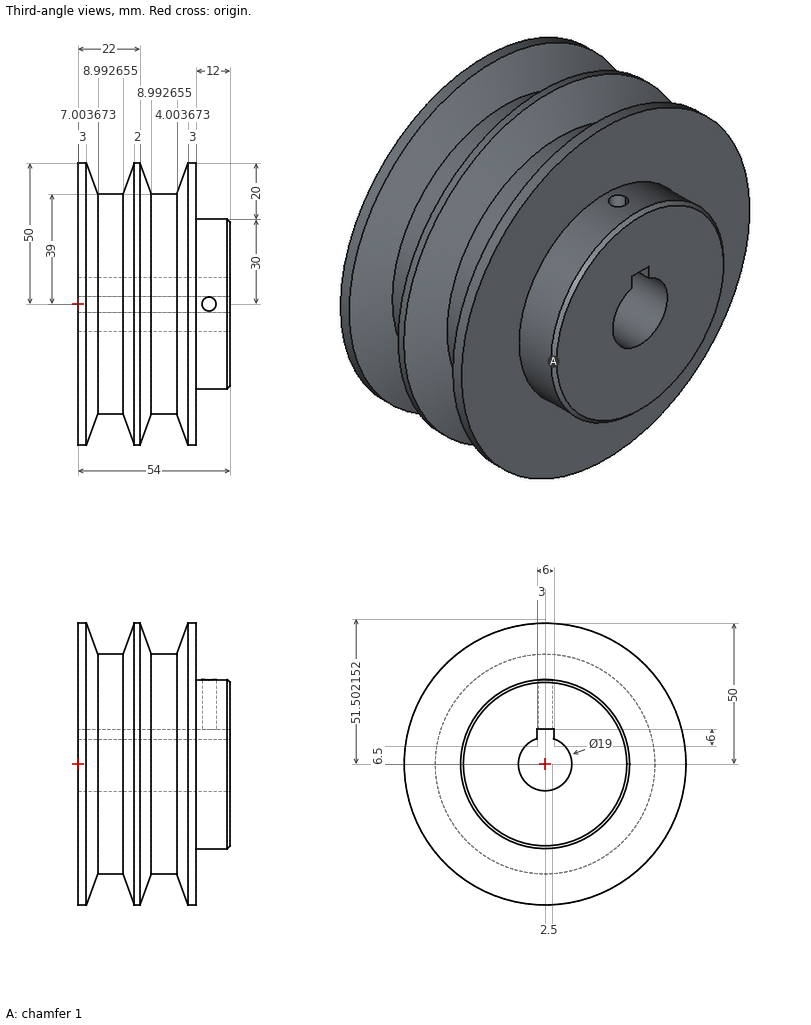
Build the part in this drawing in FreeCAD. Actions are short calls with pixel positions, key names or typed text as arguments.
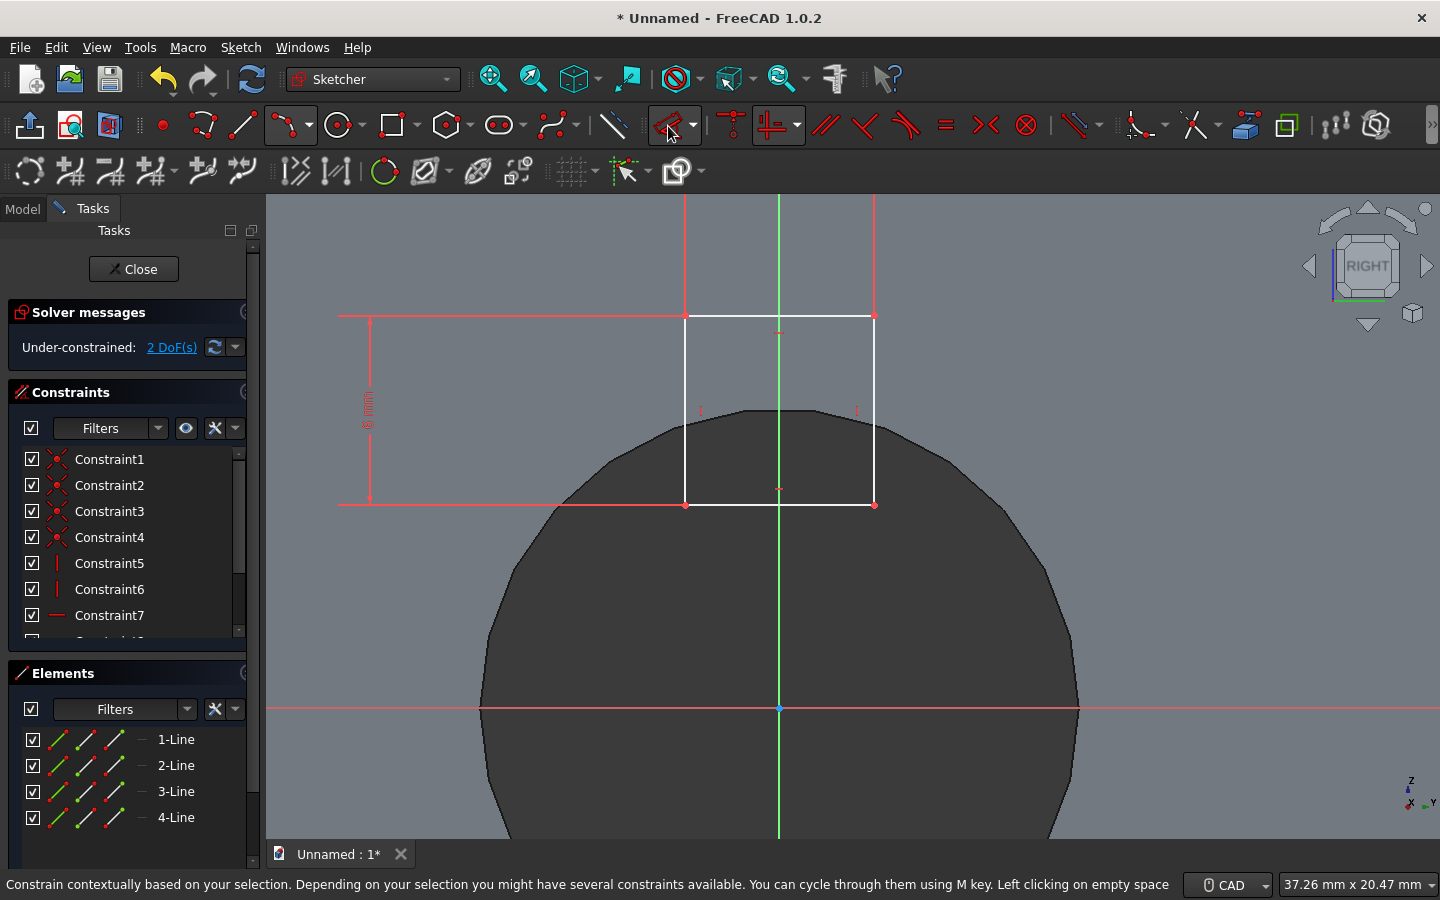
click(685, 316)
click(732, 742)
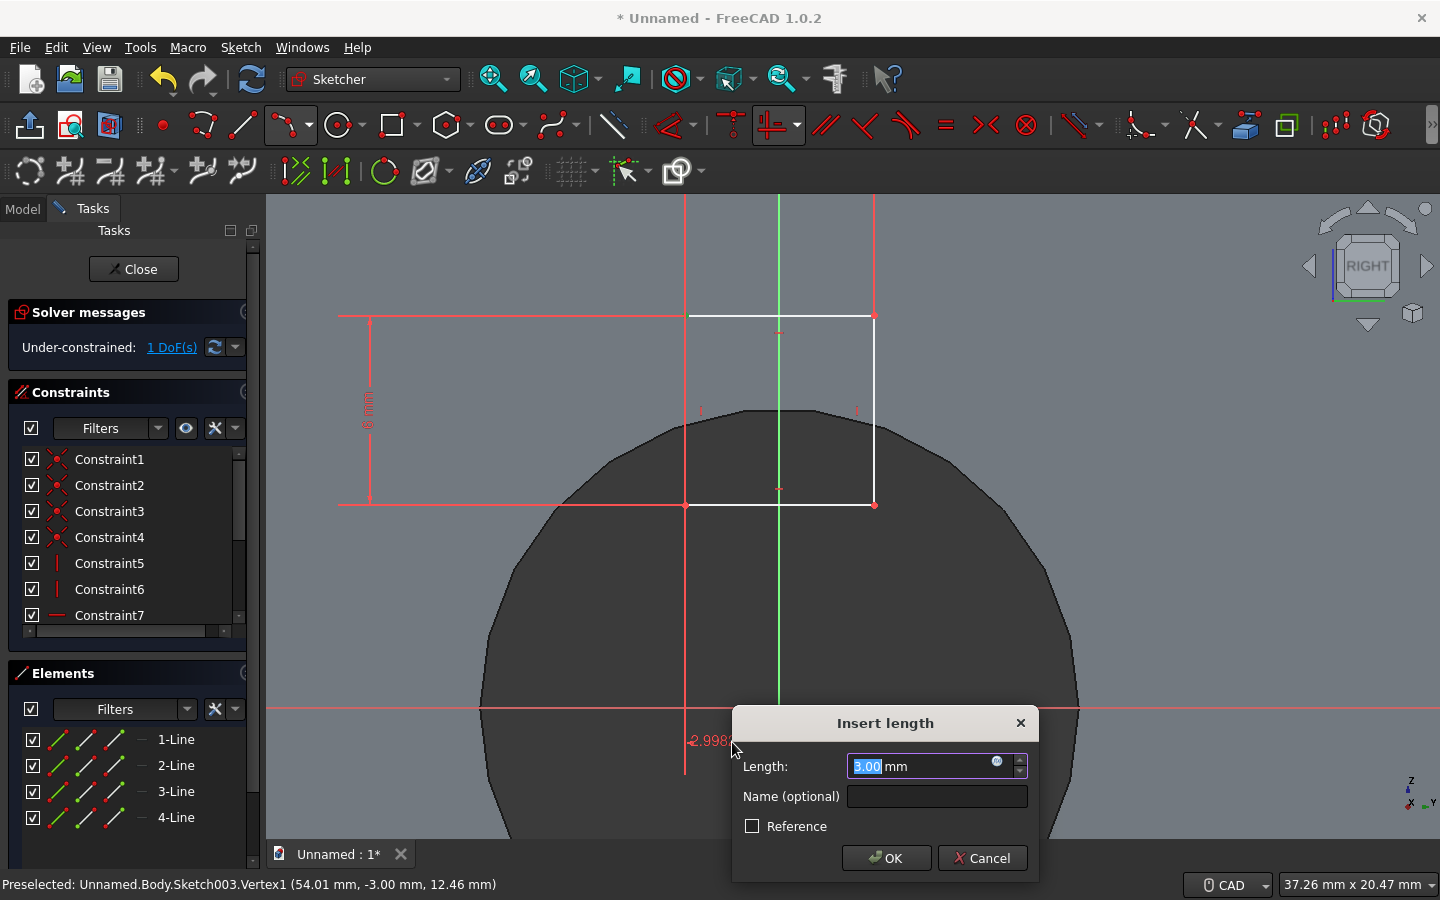
text(3)
key(Return)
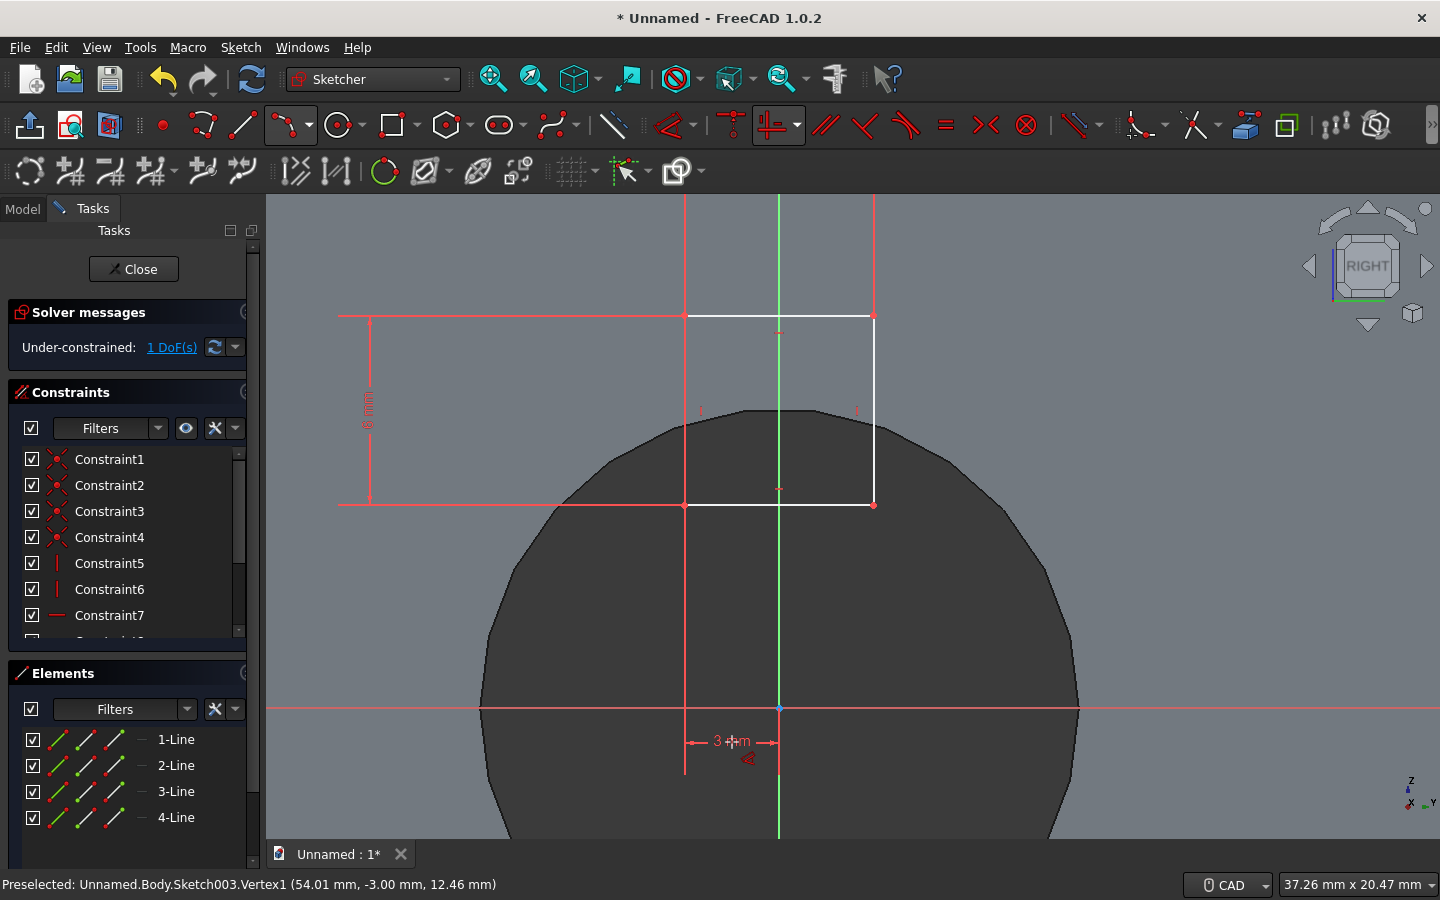
click(685, 505)
click(651, 607)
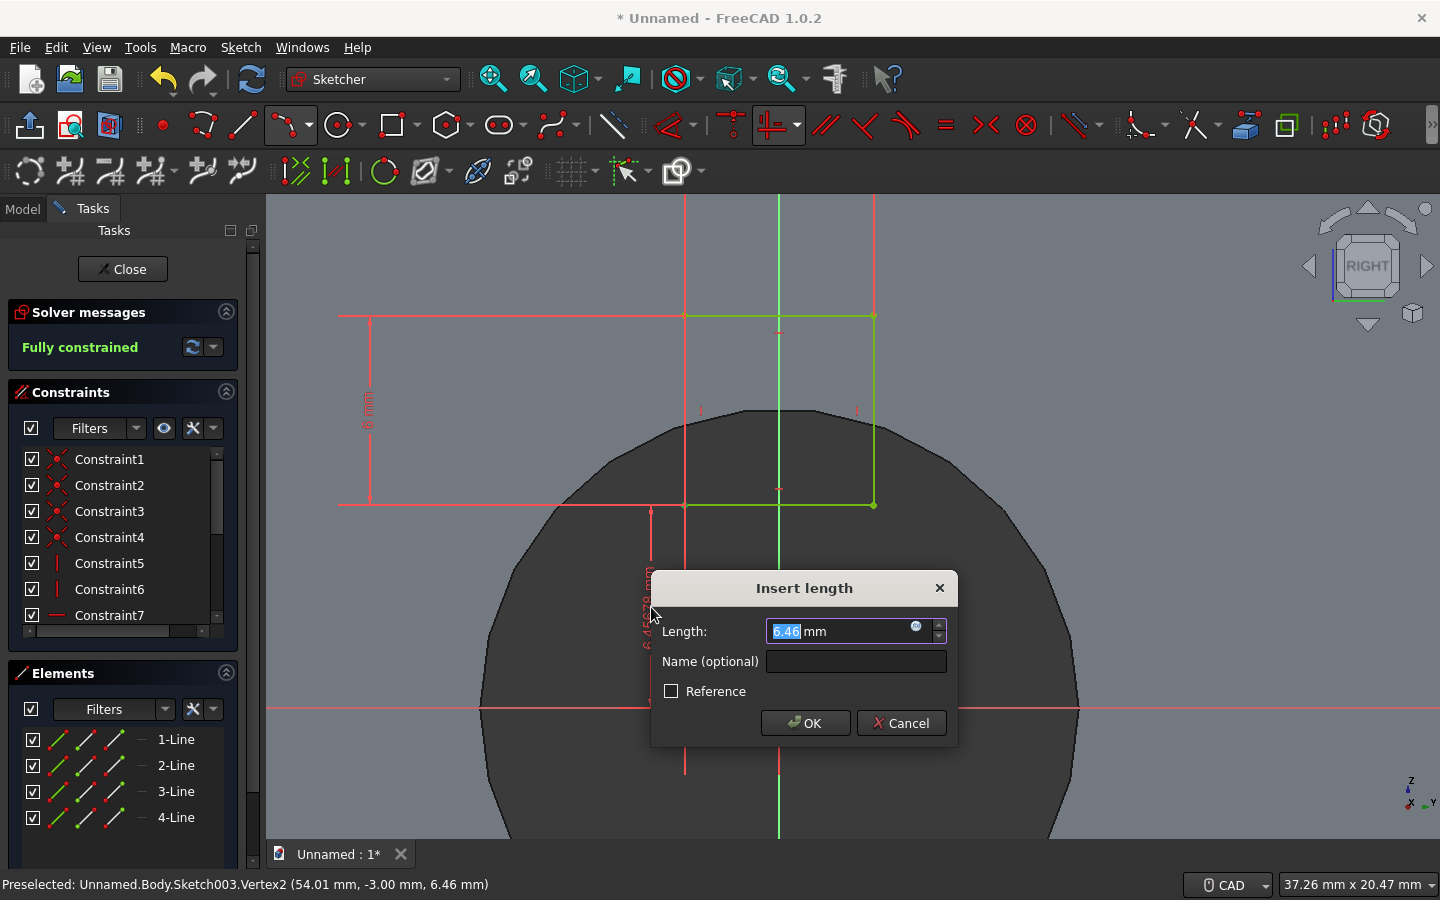
text(6.5)
key(Return)
key(Escape)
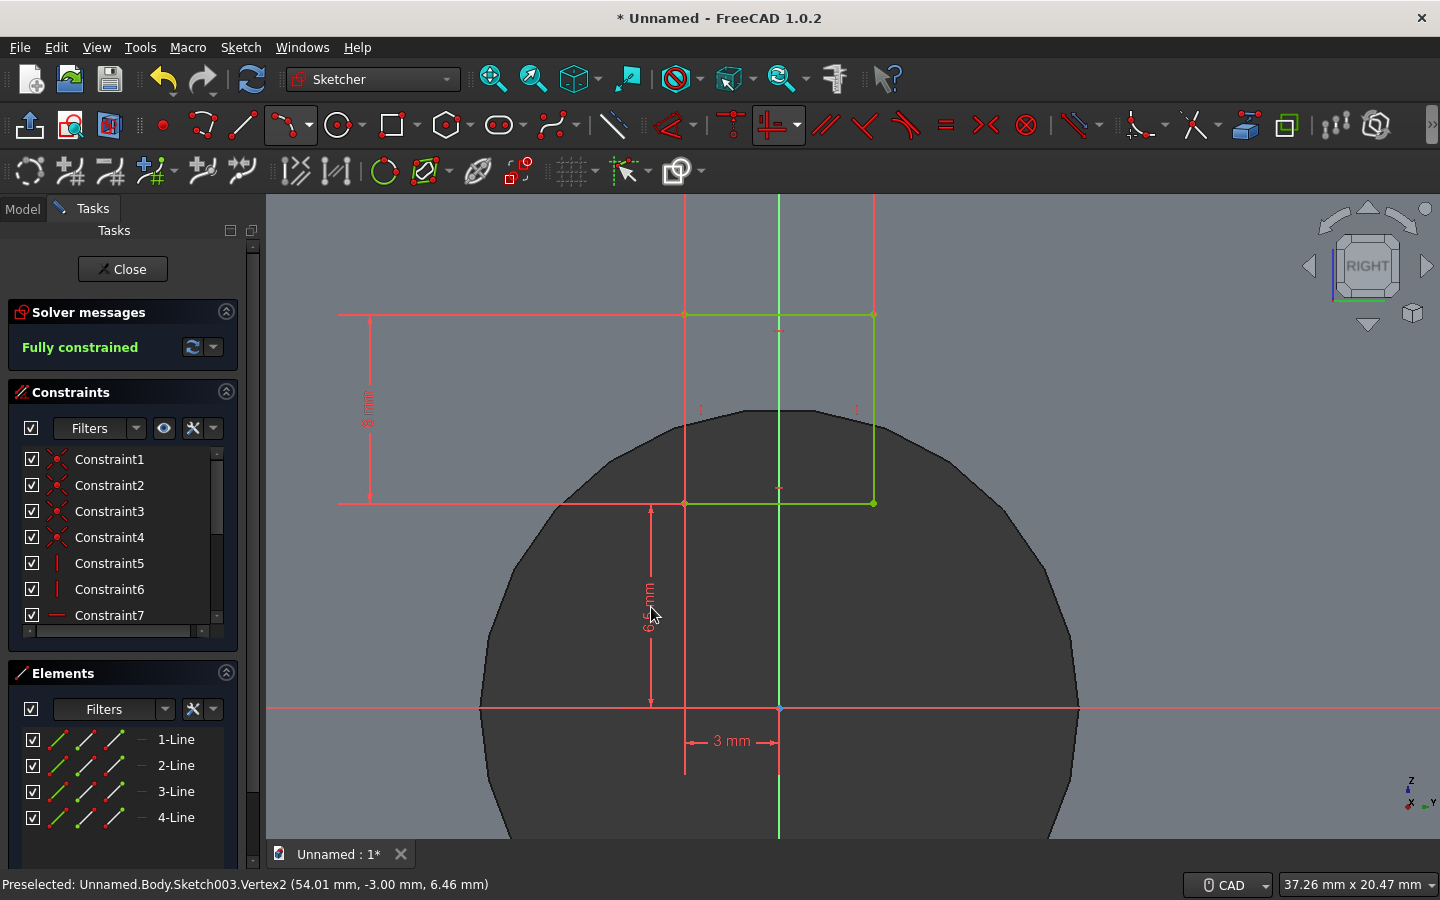
click(123, 269)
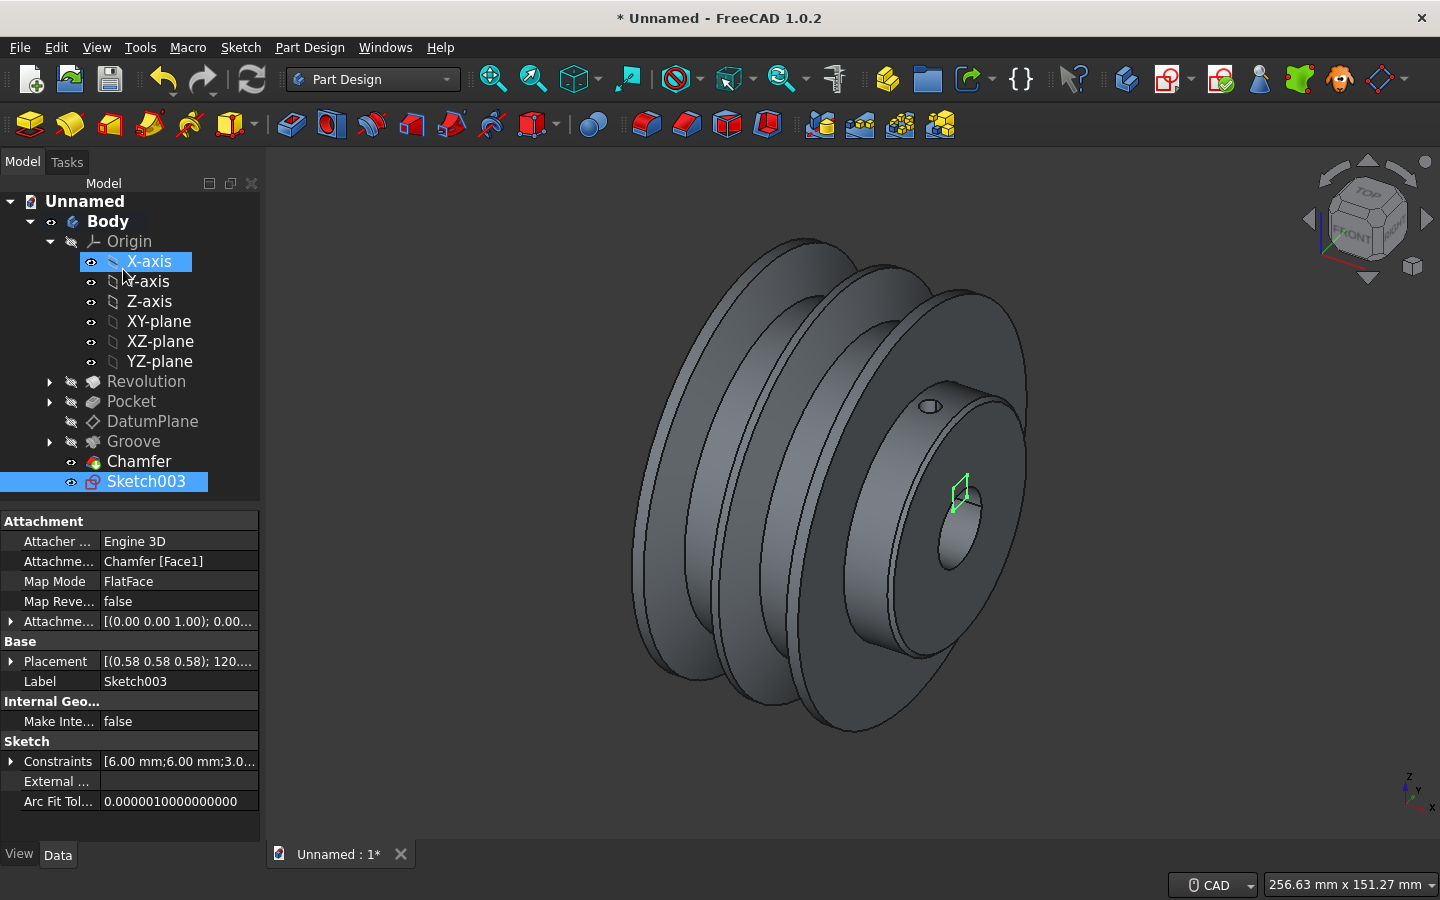
click(292, 124)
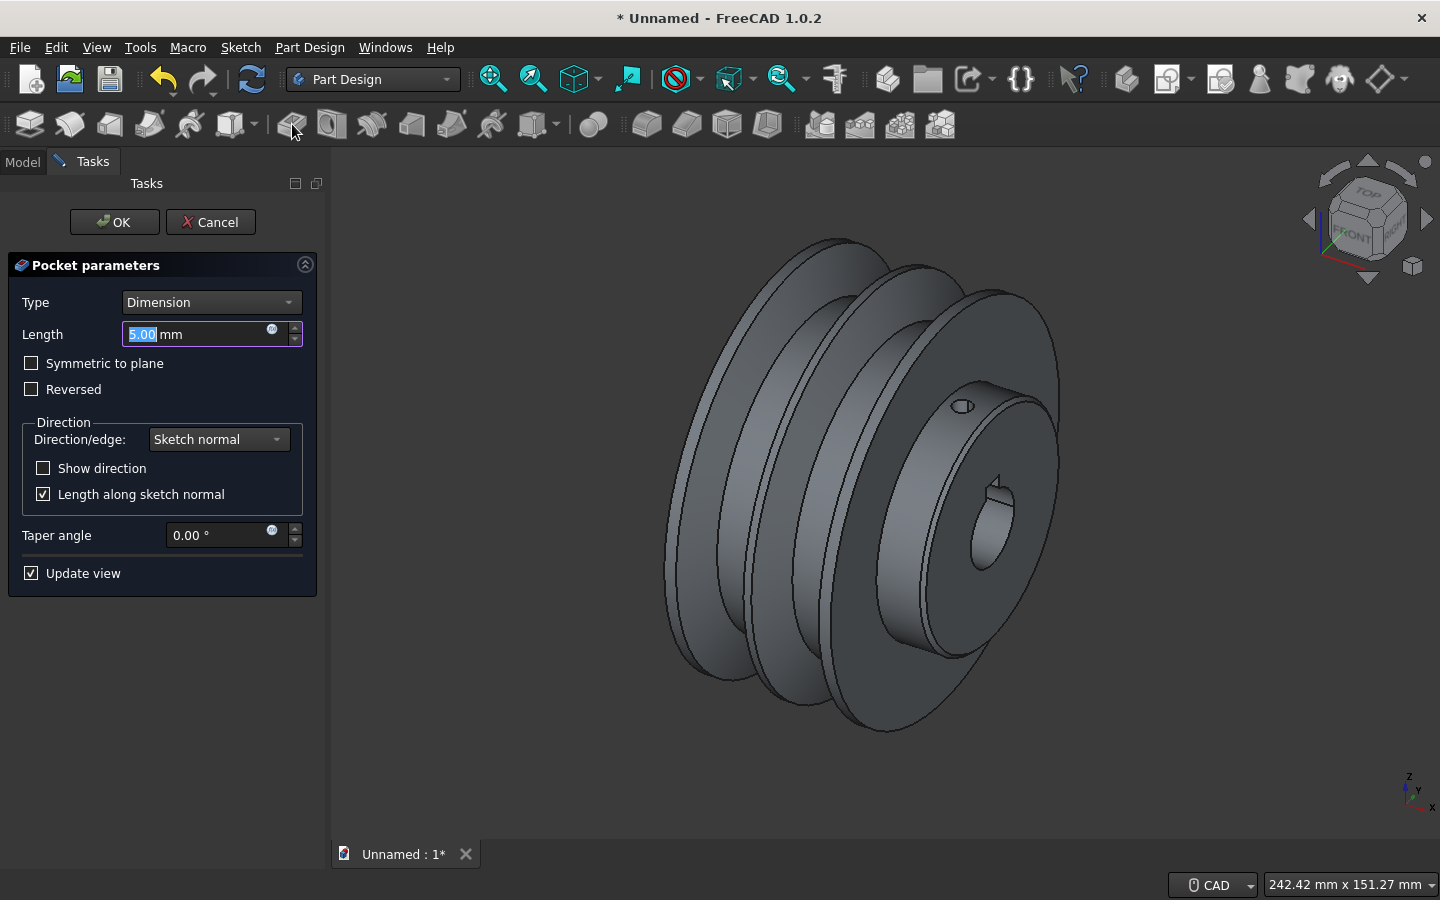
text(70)
key(Tab)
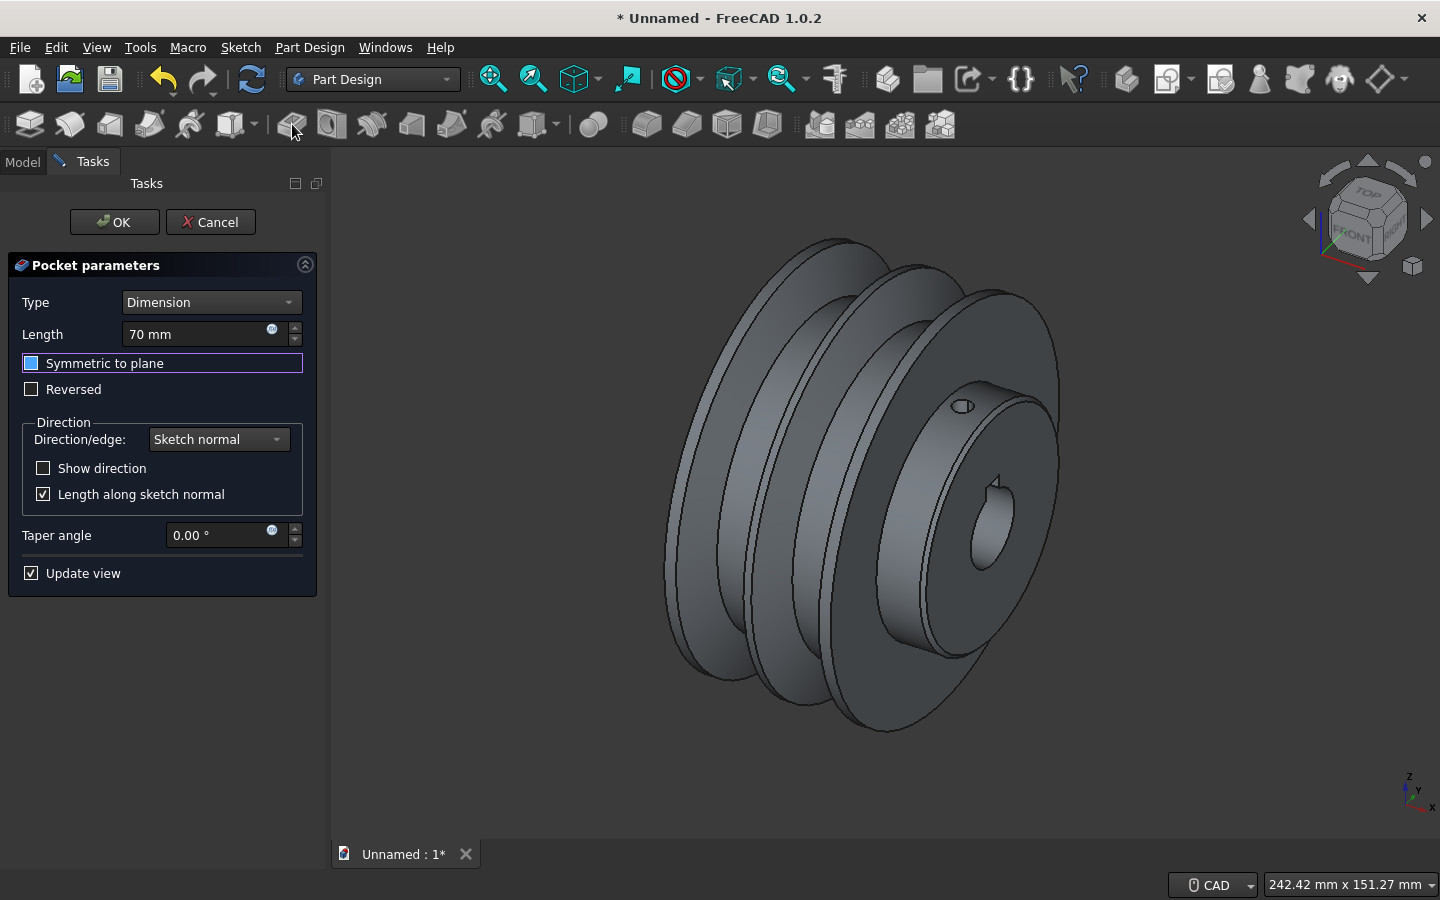
click(115, 222)